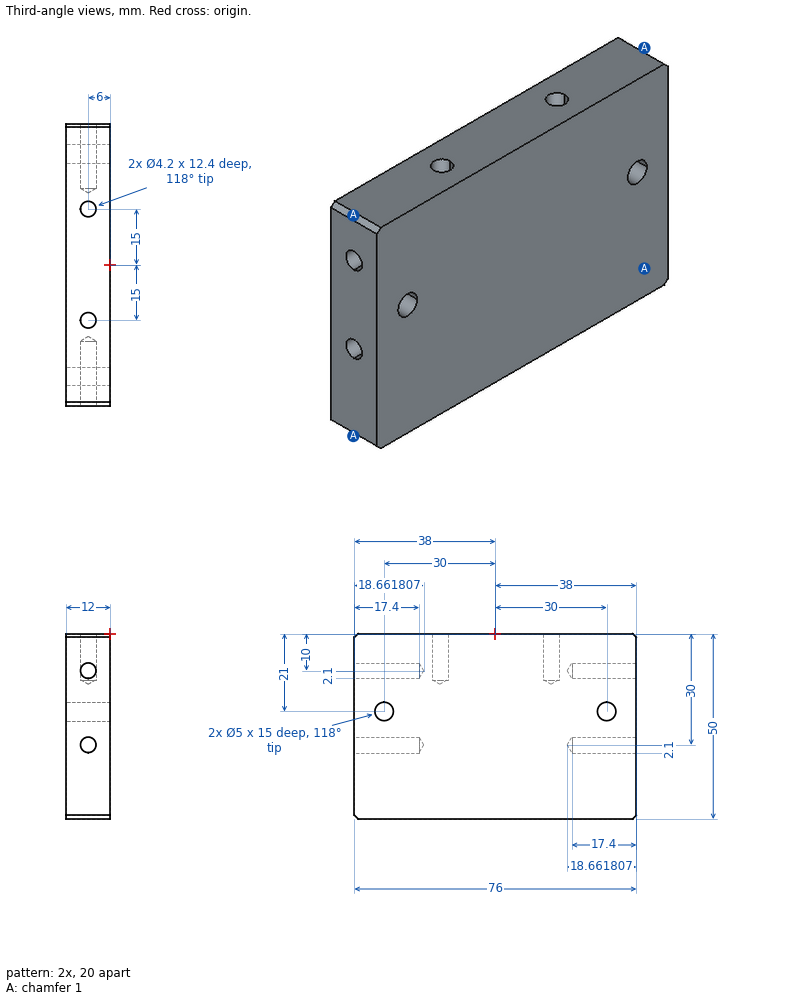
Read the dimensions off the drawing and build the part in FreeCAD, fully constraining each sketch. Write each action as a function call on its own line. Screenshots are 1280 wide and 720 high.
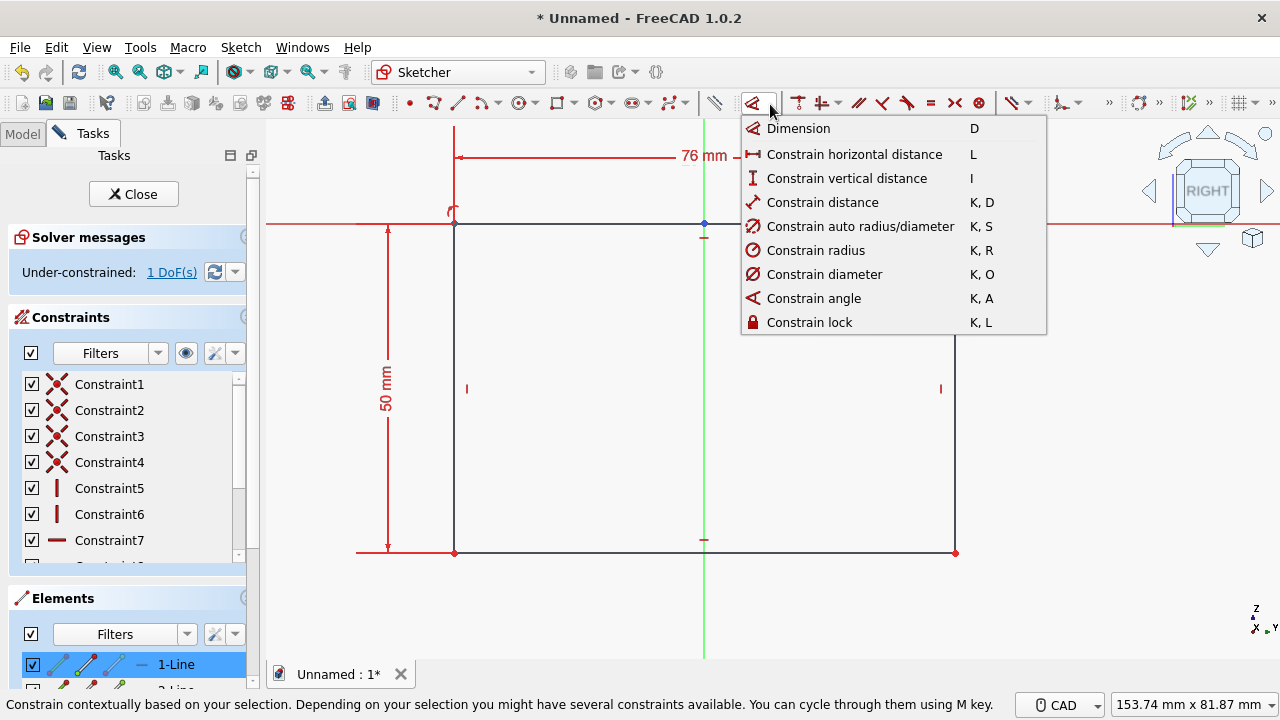
click(894, 154)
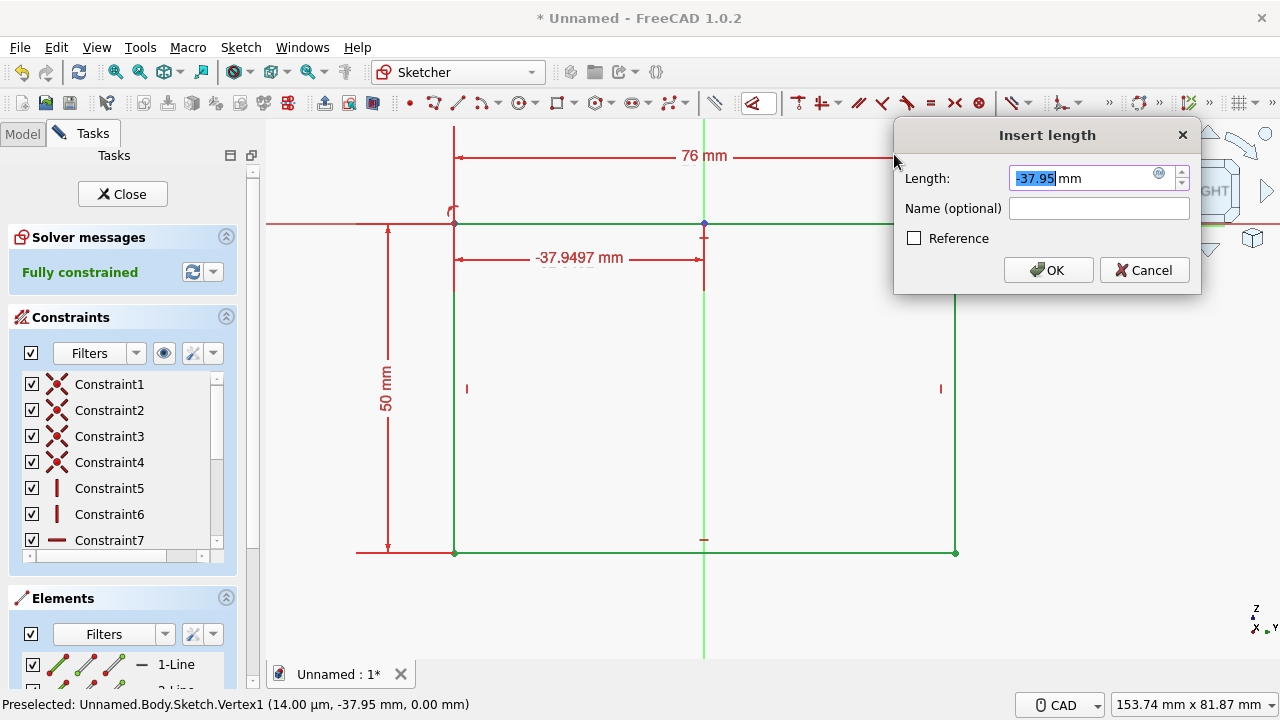
text(-38)
key(Return)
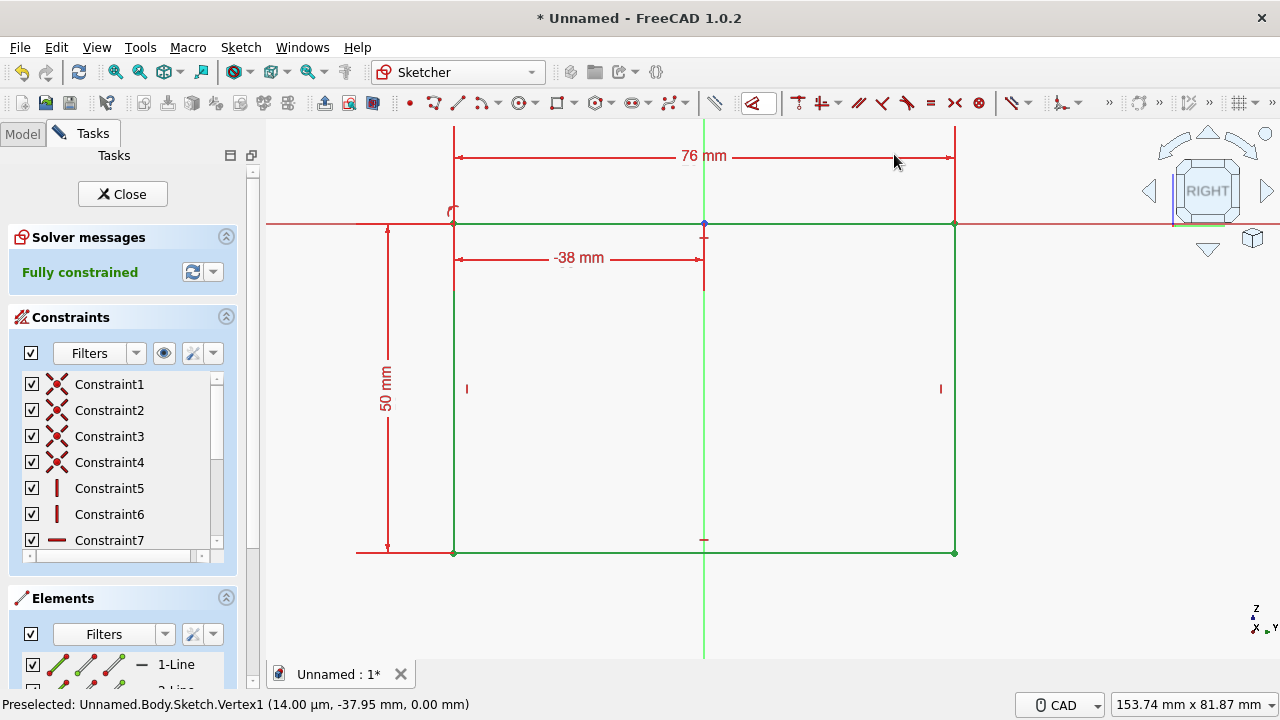
click(123, 194)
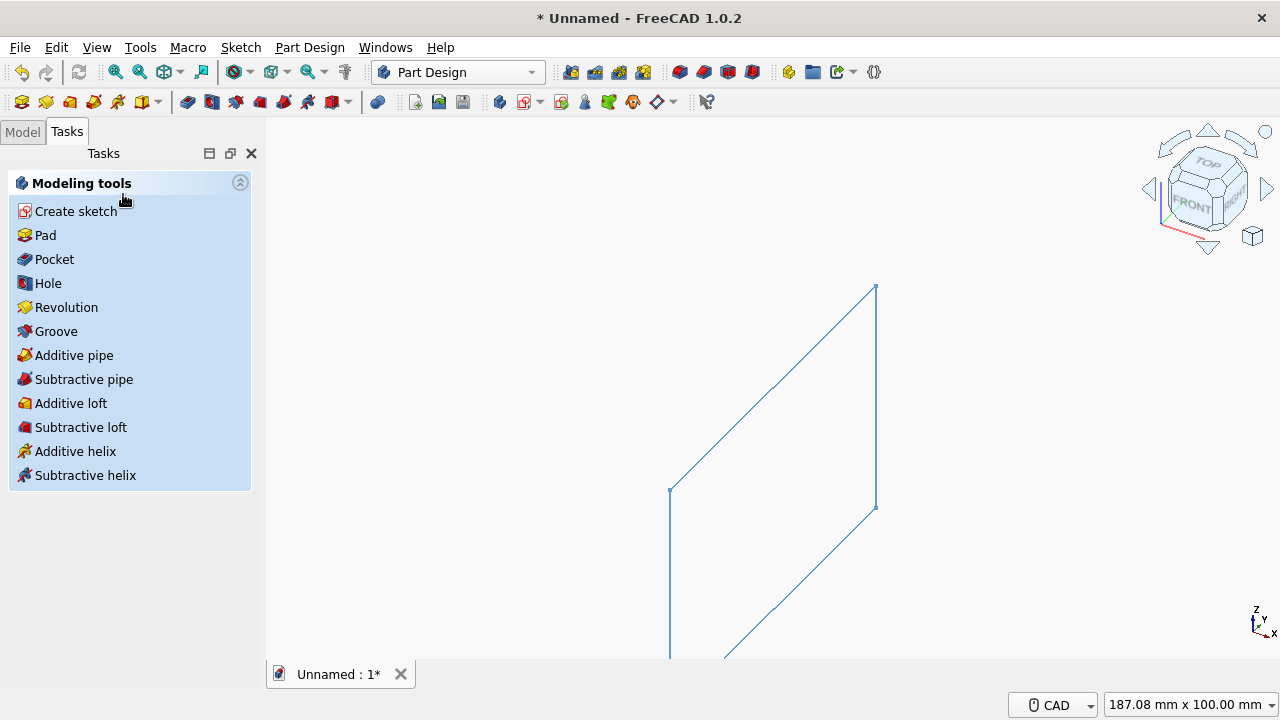
click(22, 102)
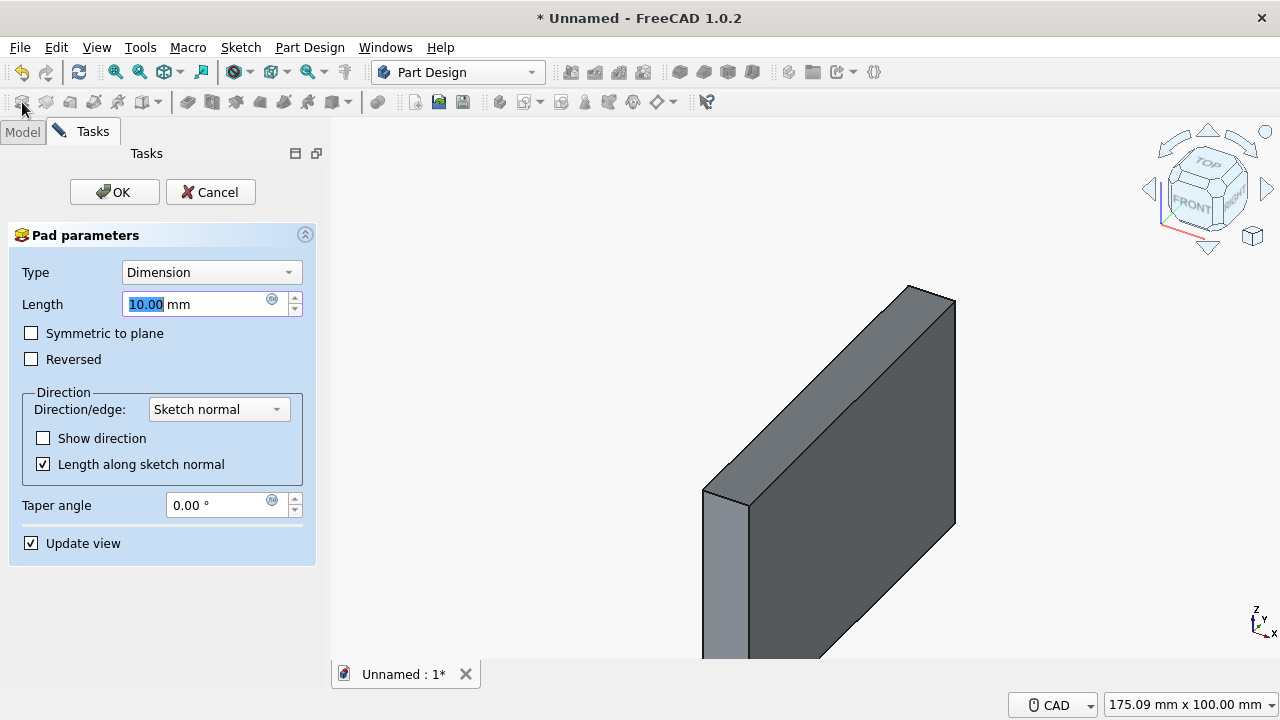
text(12)
key(Tab)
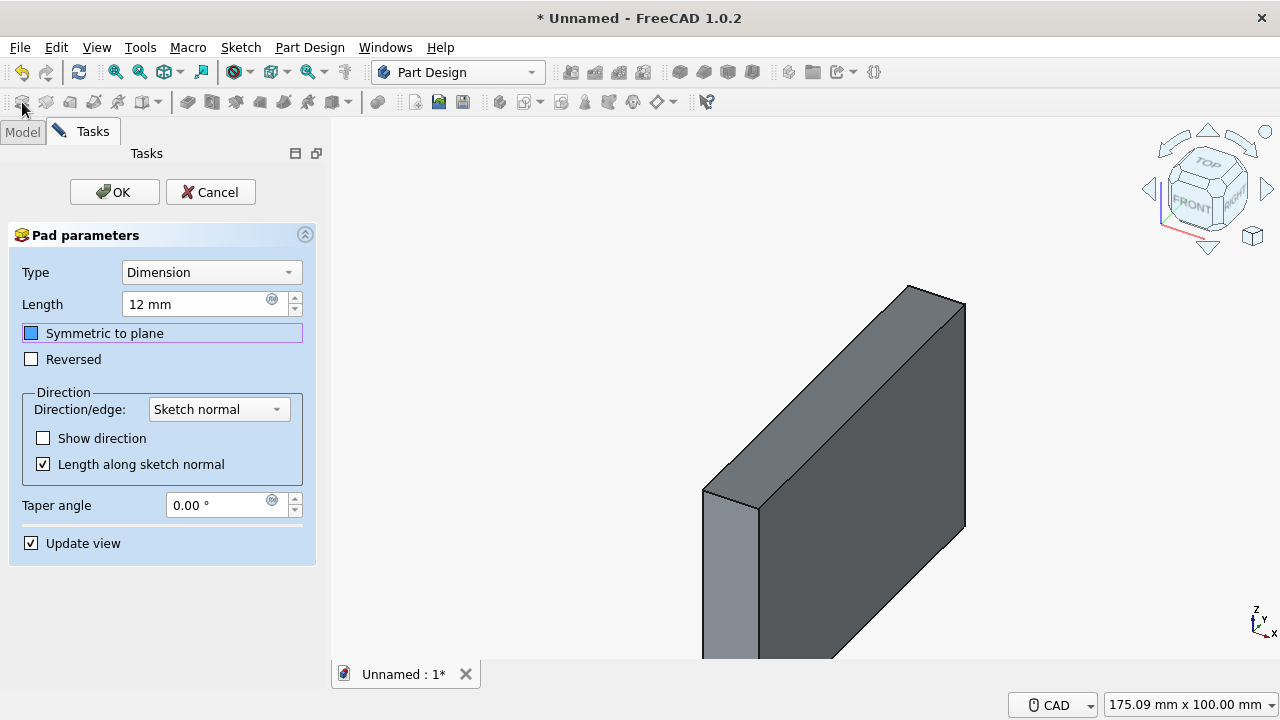
click(30, 359)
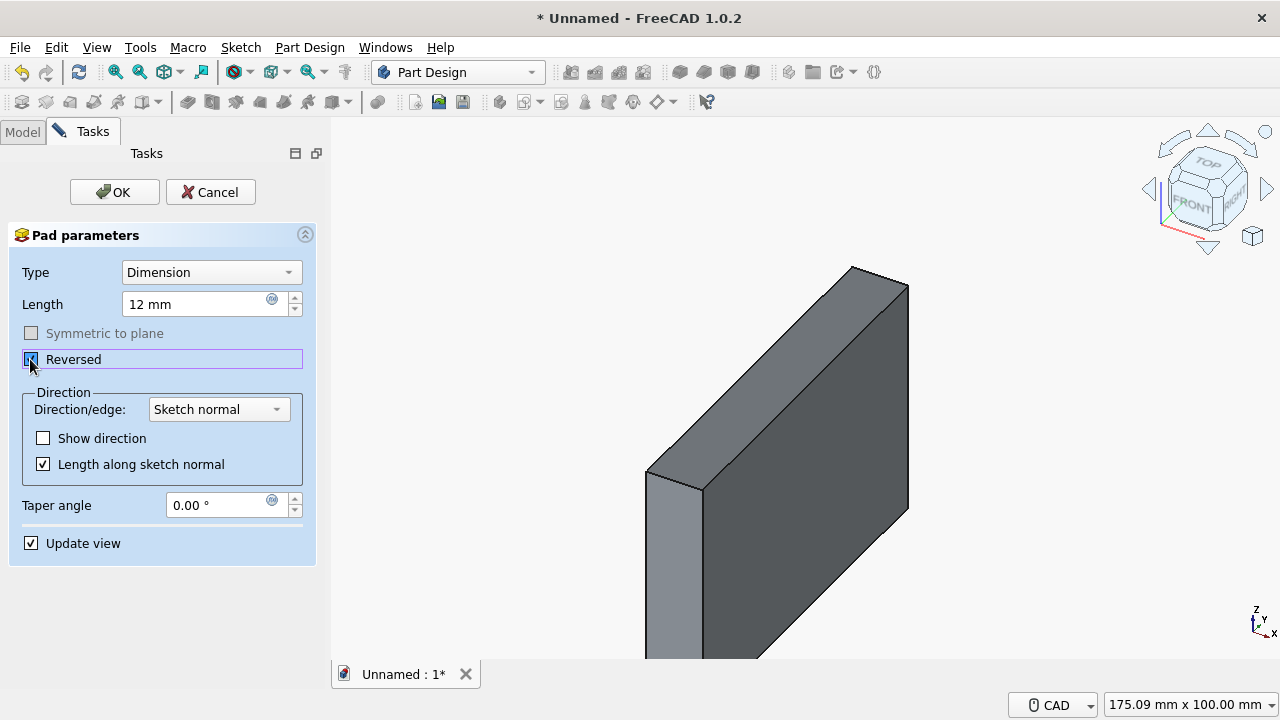
click(115, 192)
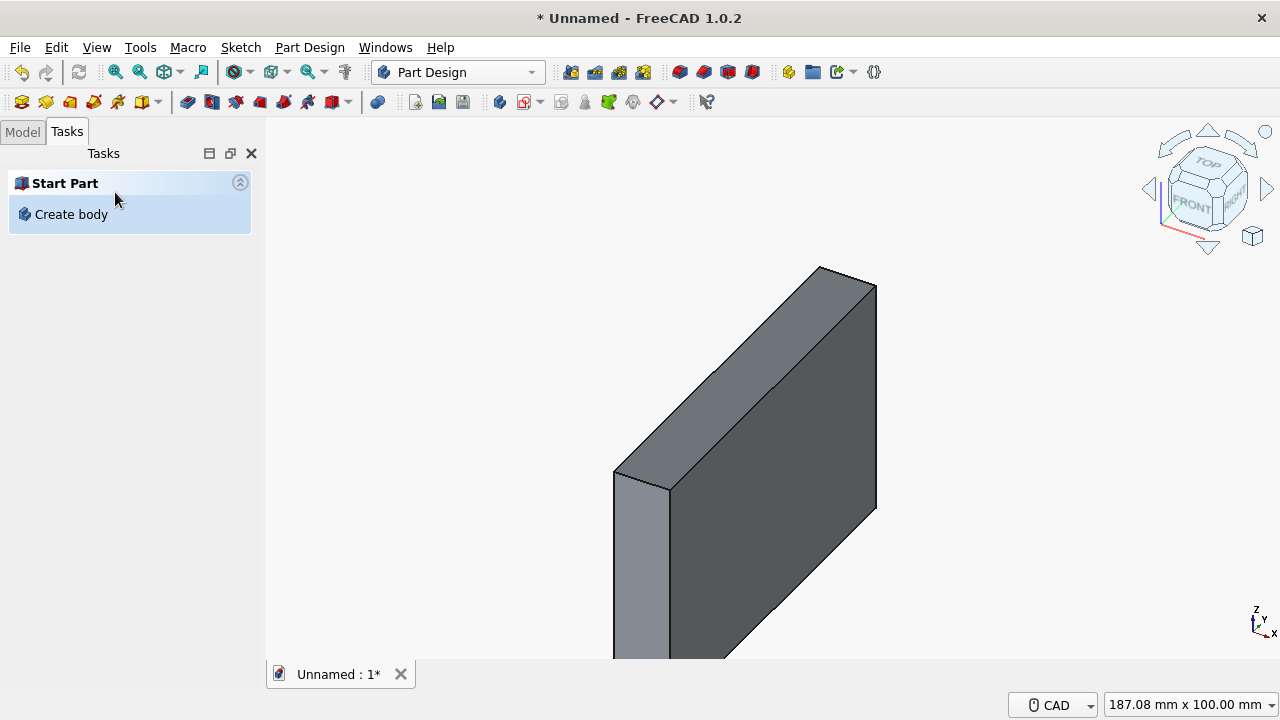
click(116, 72)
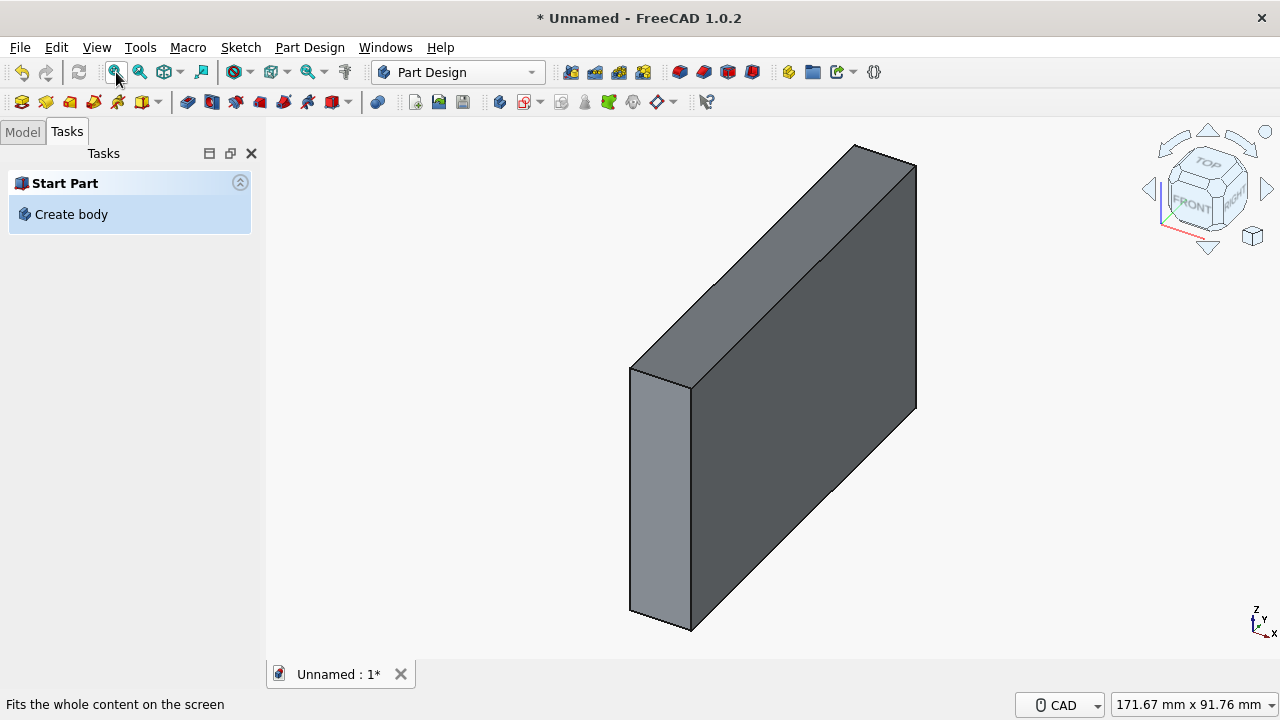
click(524, 102)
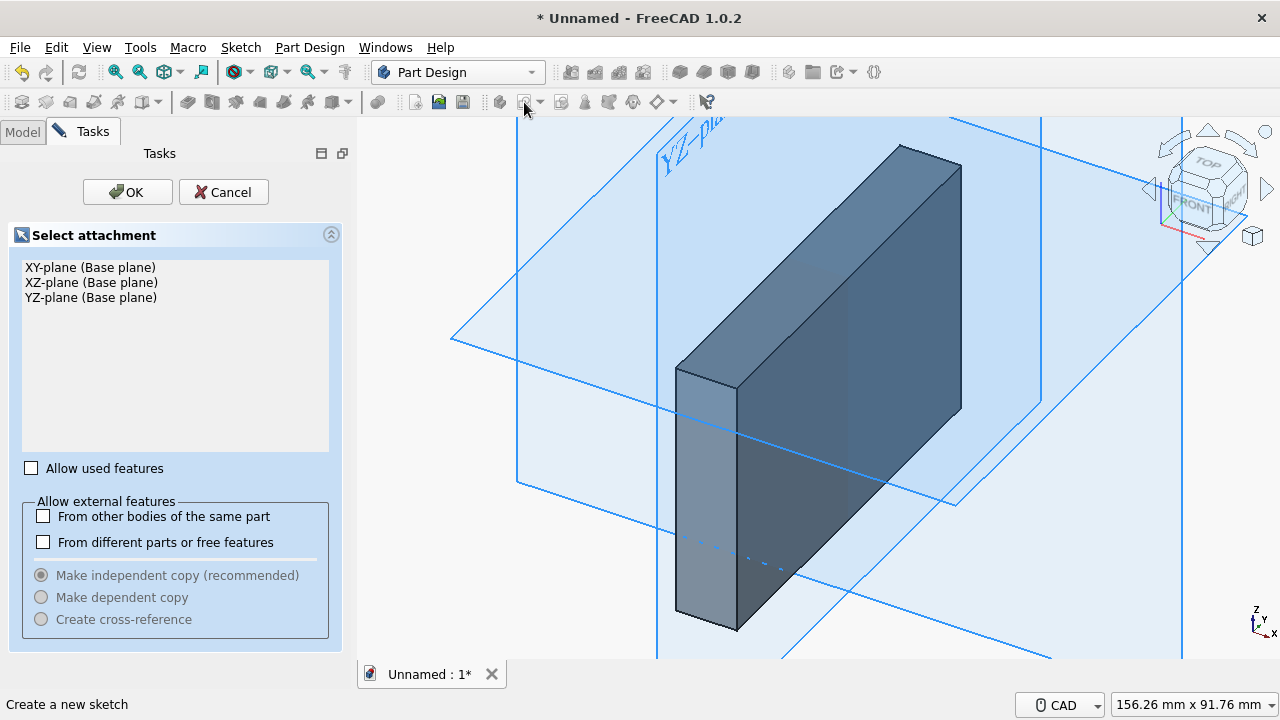
click(82, 298)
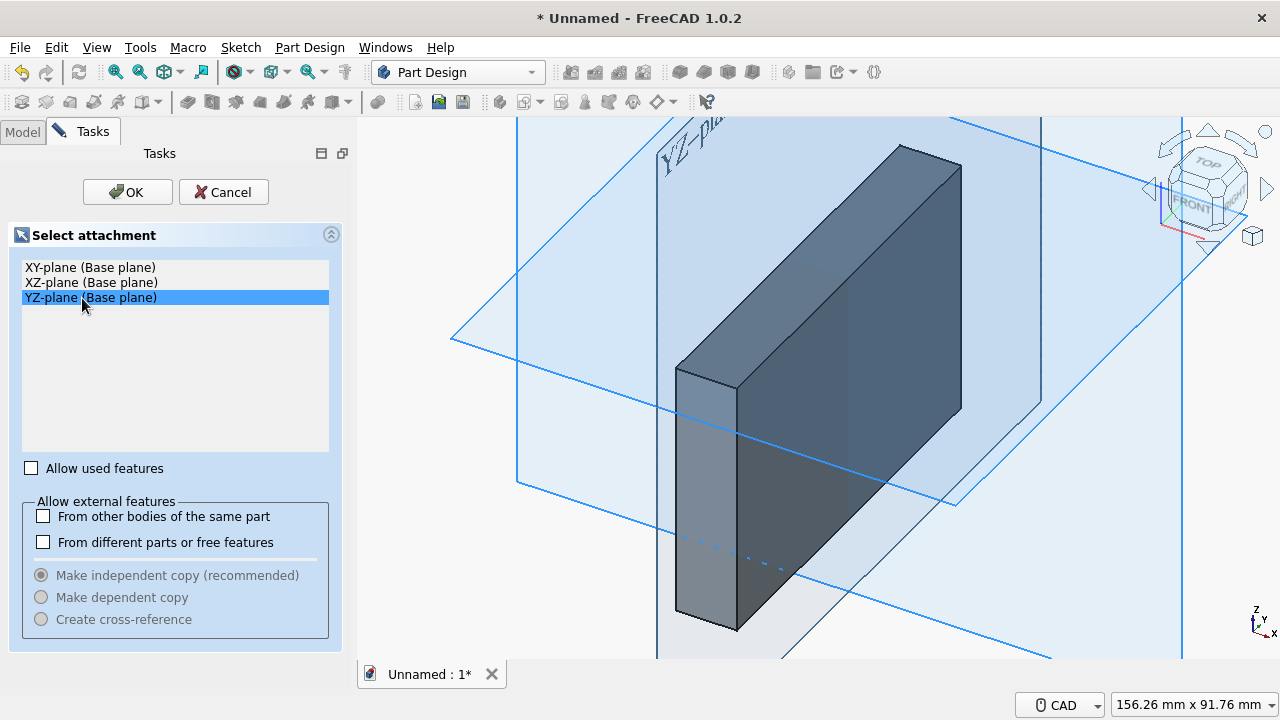
click(128, 192)